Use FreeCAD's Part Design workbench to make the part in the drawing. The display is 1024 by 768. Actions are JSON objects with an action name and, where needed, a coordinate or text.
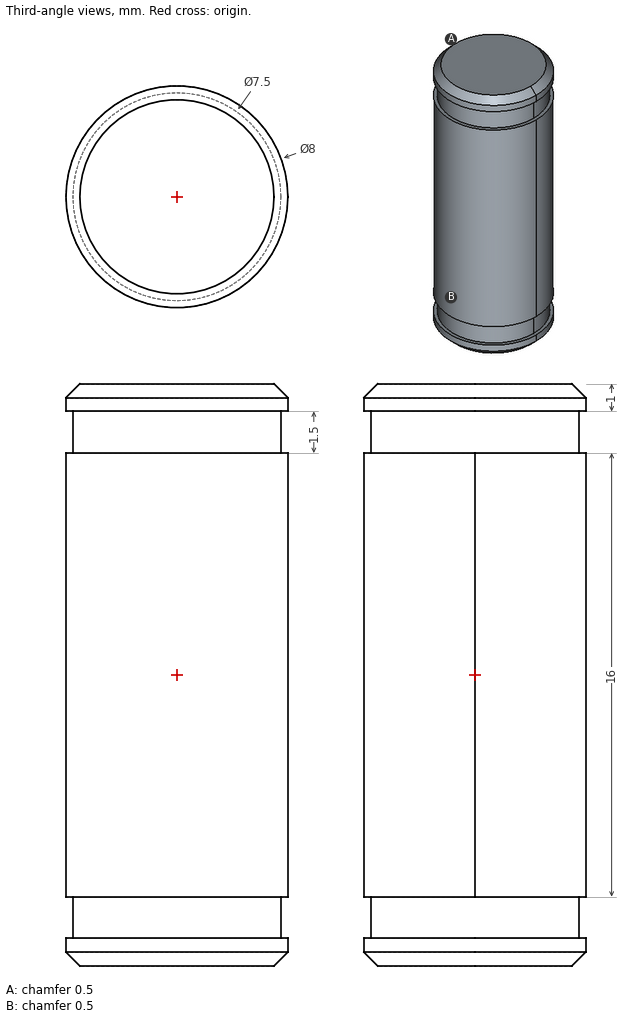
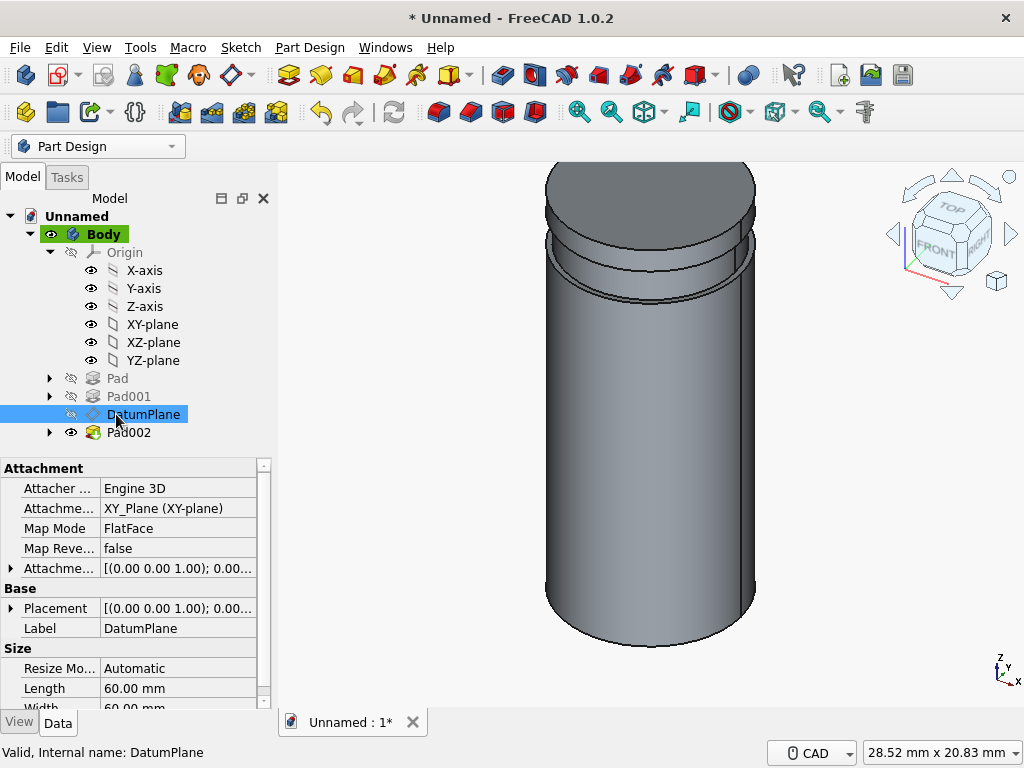
{"action": "key", "text": "v f"}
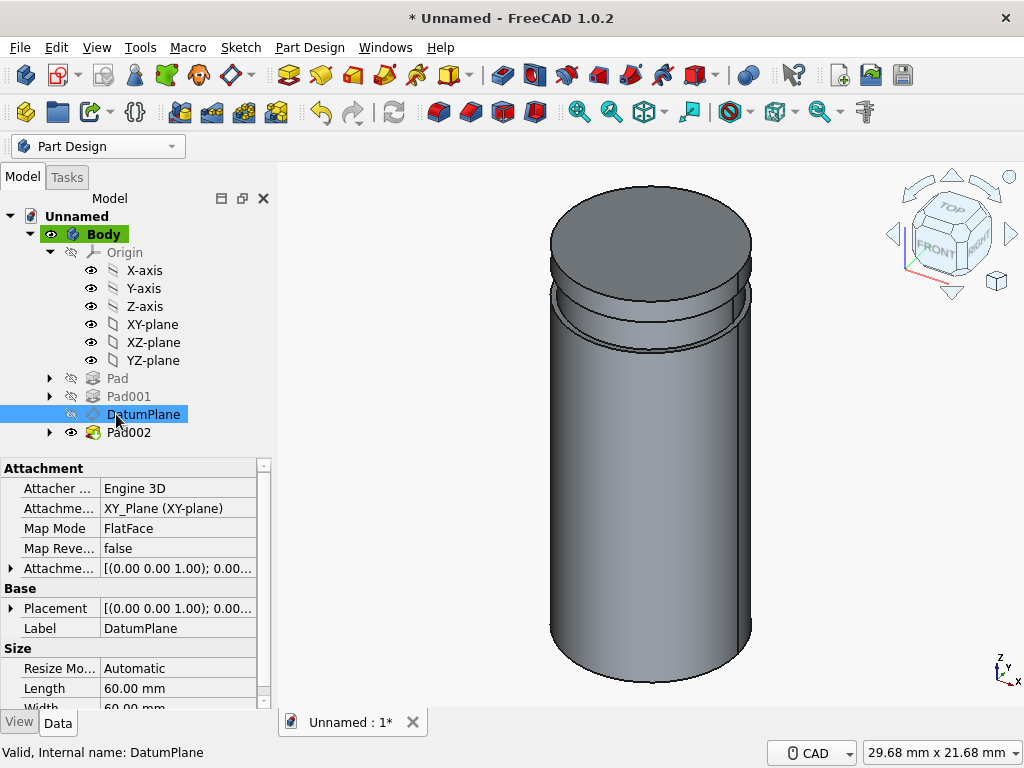
{"action": "left_click", "coordinate": [551, 249]}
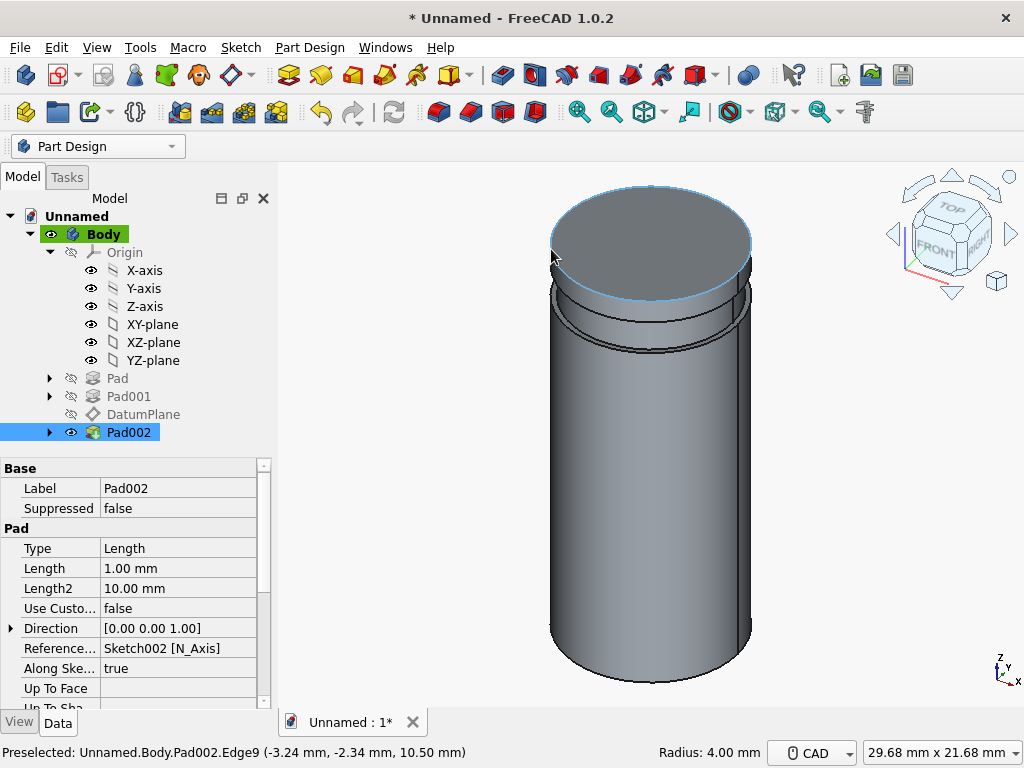
{"action": "left_click", "coordinate": [472, 112]}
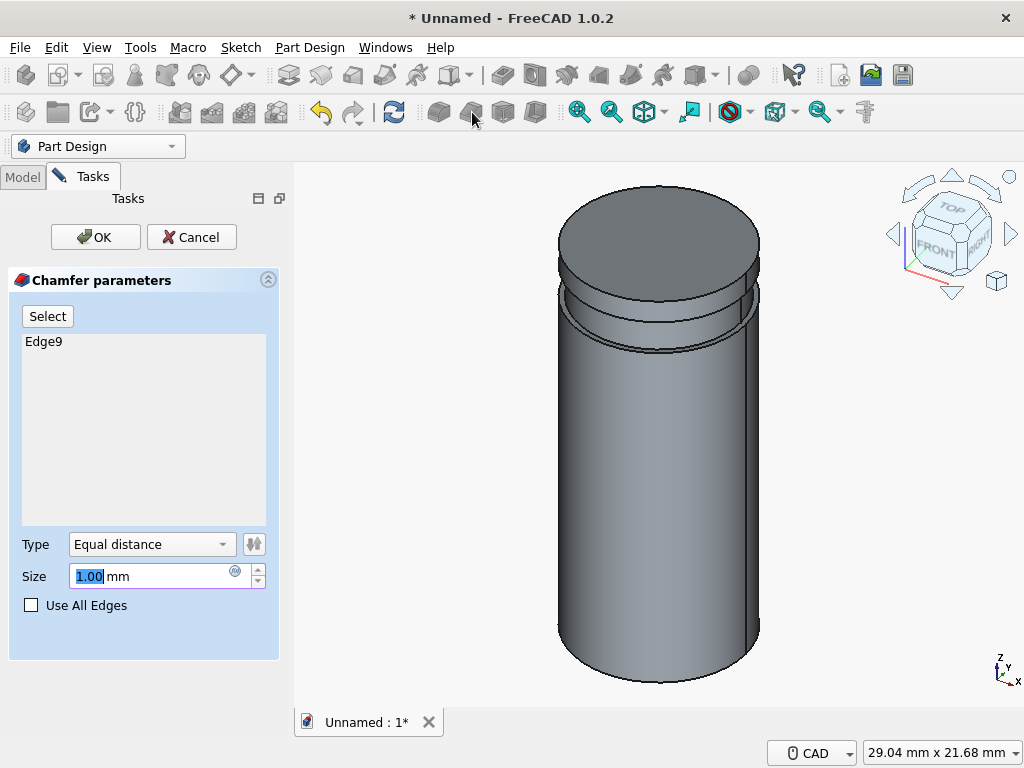
{"action": "type", "text": "0.5"}
{"action": "key", "text": "Tab"}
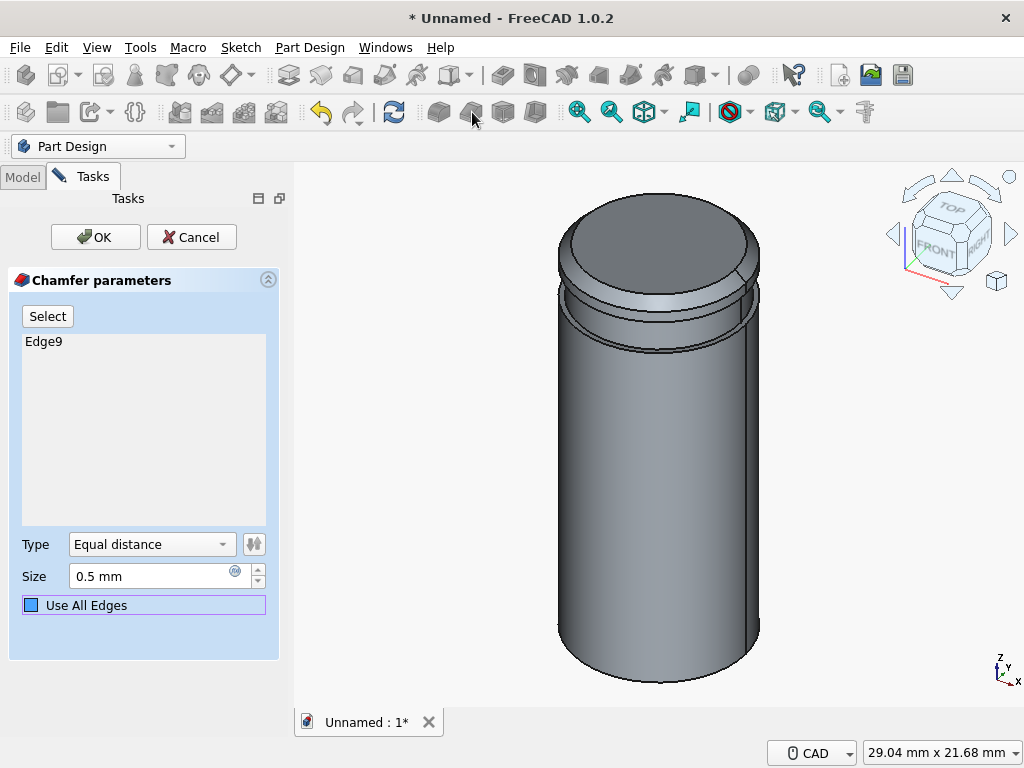
{"action": "left_click", "coordinate": [96, 237]}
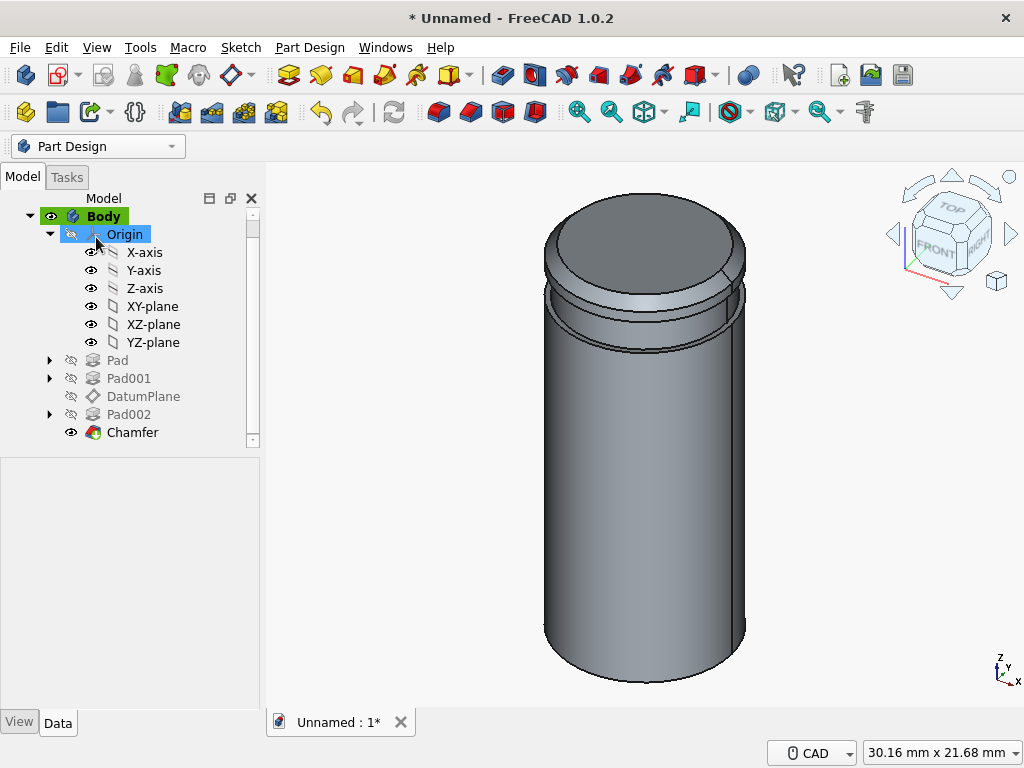
{"action": "left_click", "coordinate": [116, 378]}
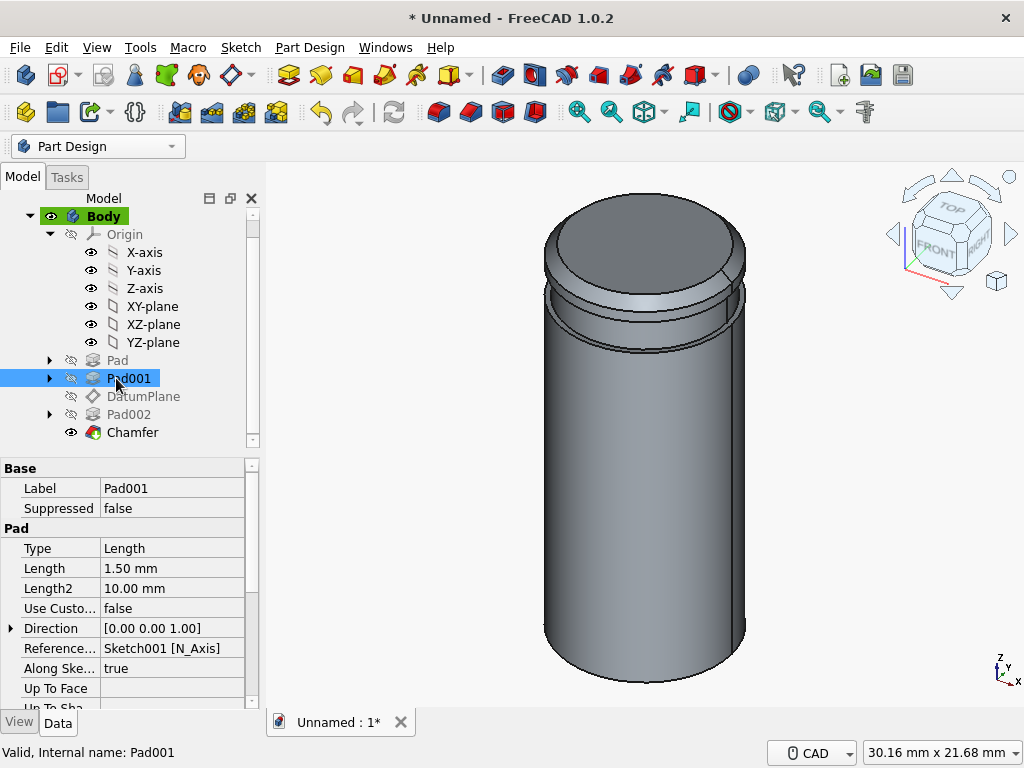
{"action": "left_click", "coordinate": [116, 414], "text": "ctrl"}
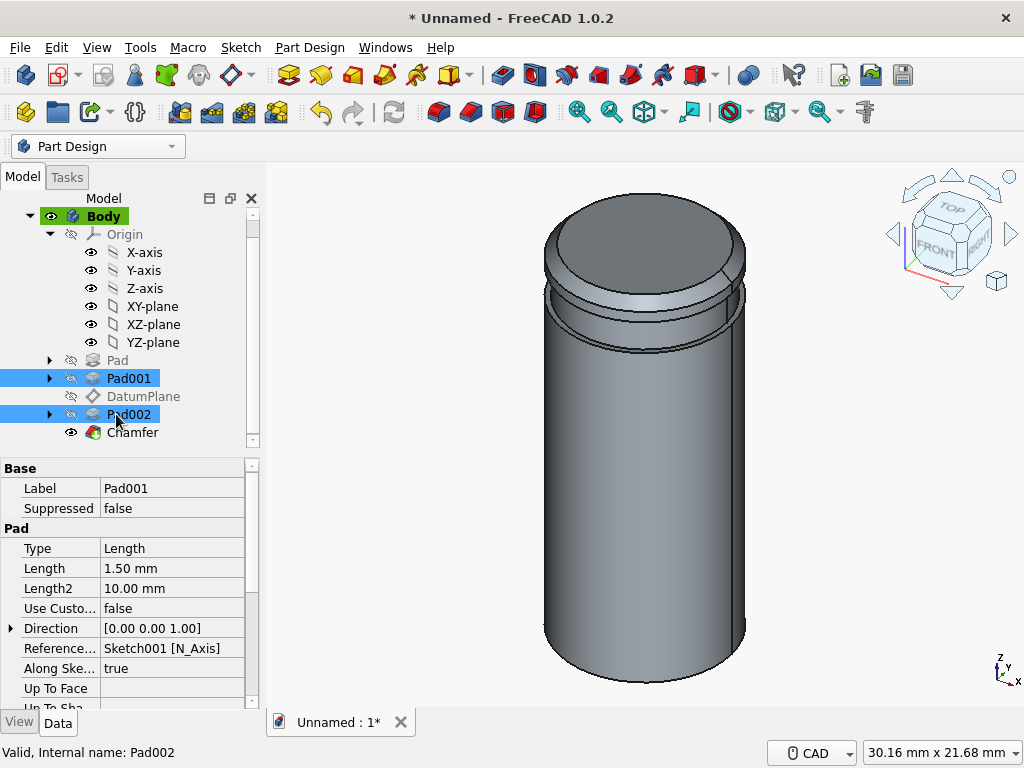
{"action": "left_click", "coordinate": [180, 112]}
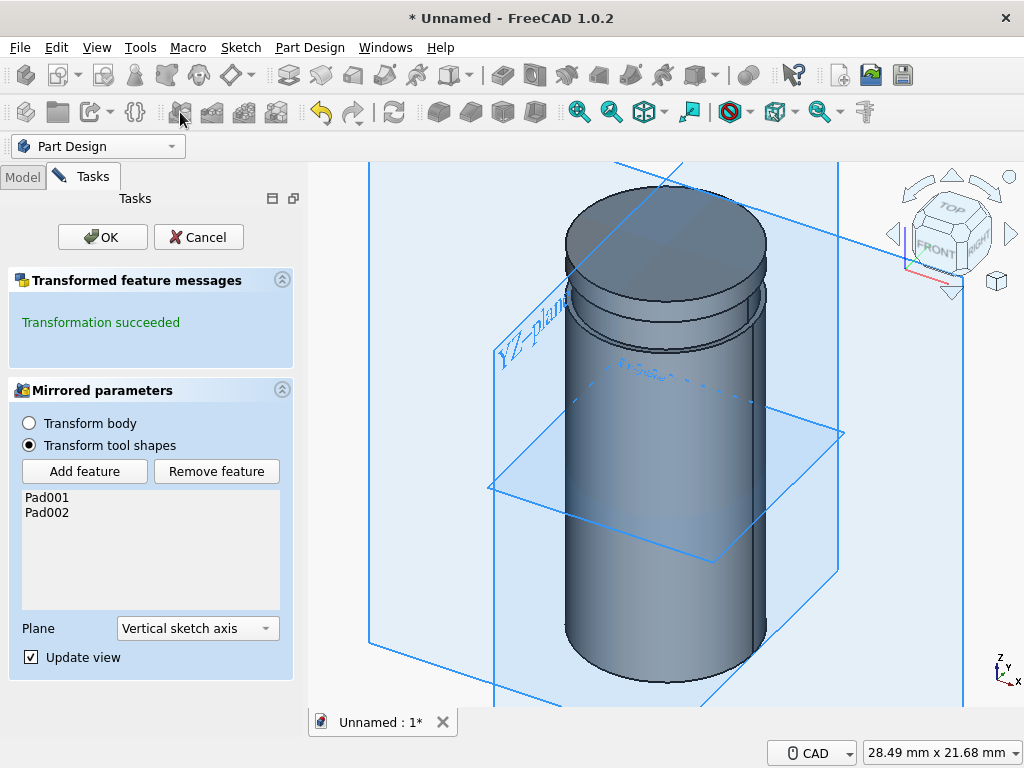
{"action": "left_click", "coordinate": [198, 628]}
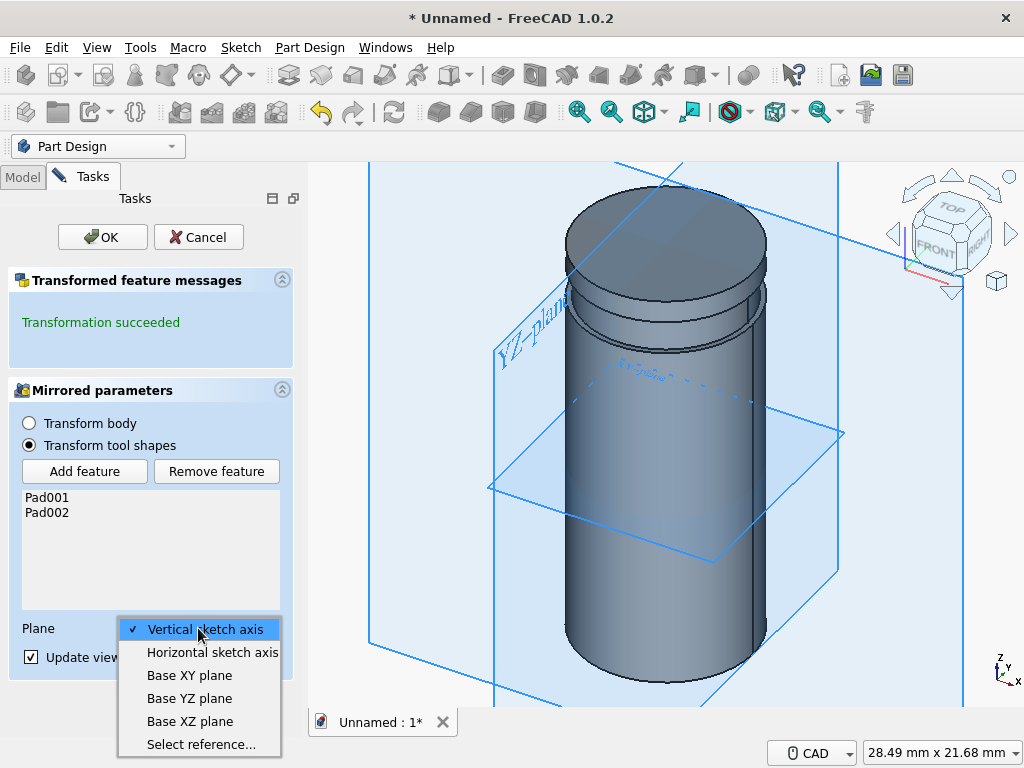
{"action": "left_click", "coordinate": [198, 676]}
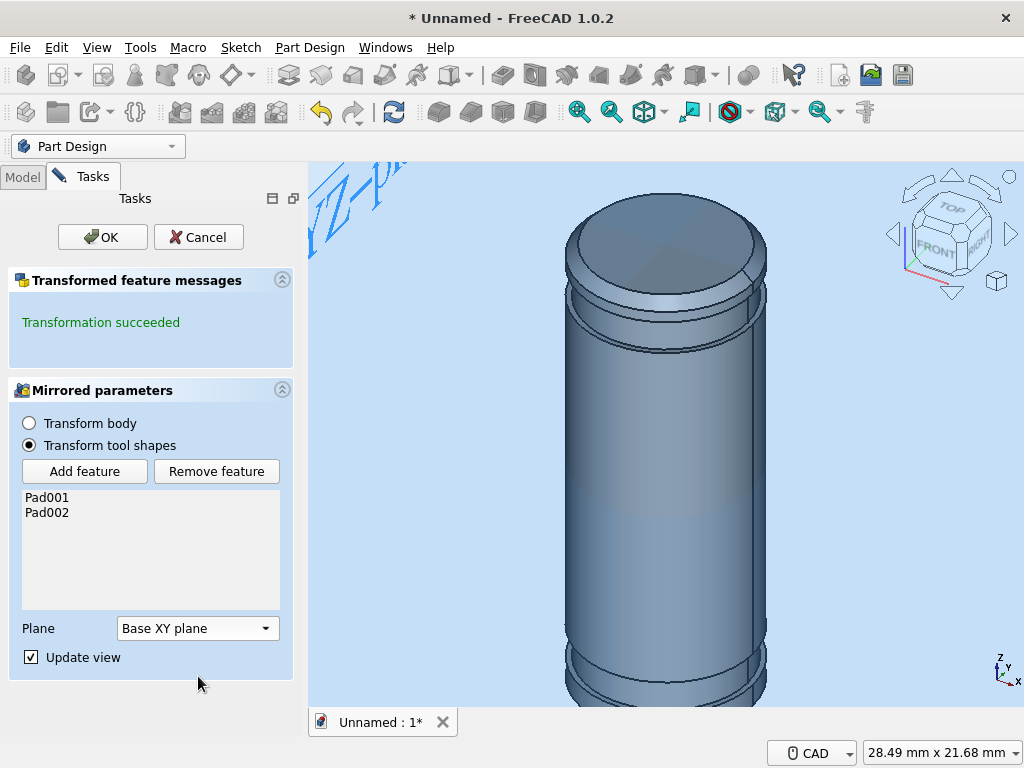
{"action": "left_click", "coordinate": [103, 237]}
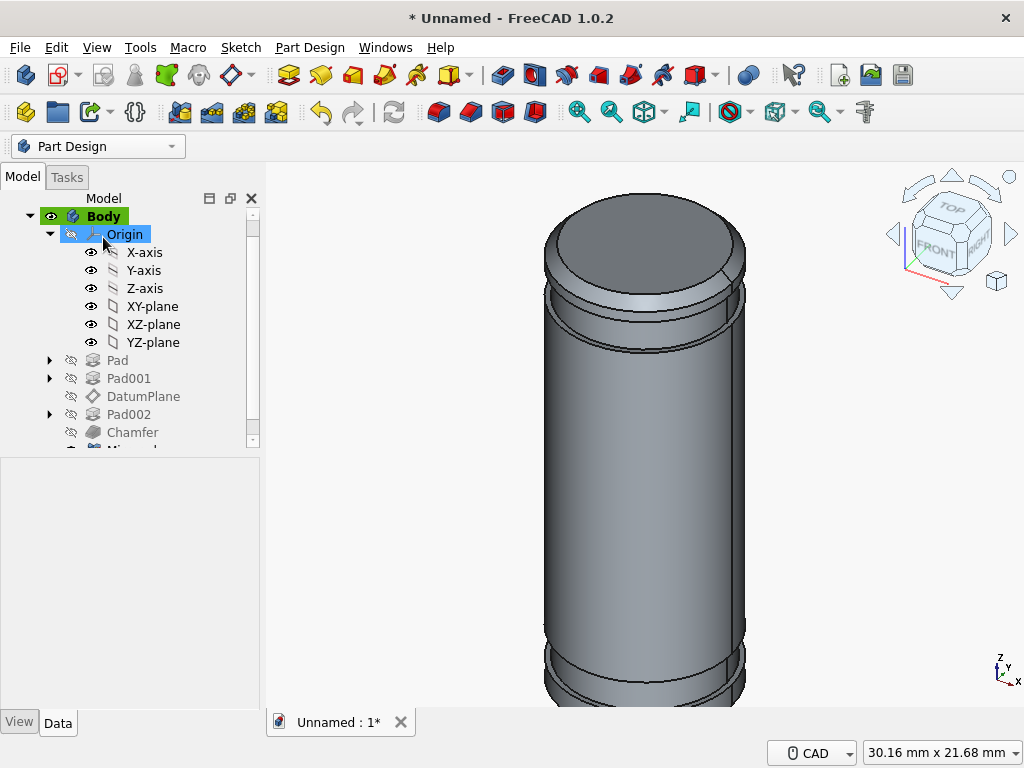
{"action": "left_click", "coordinate": [580, 112]}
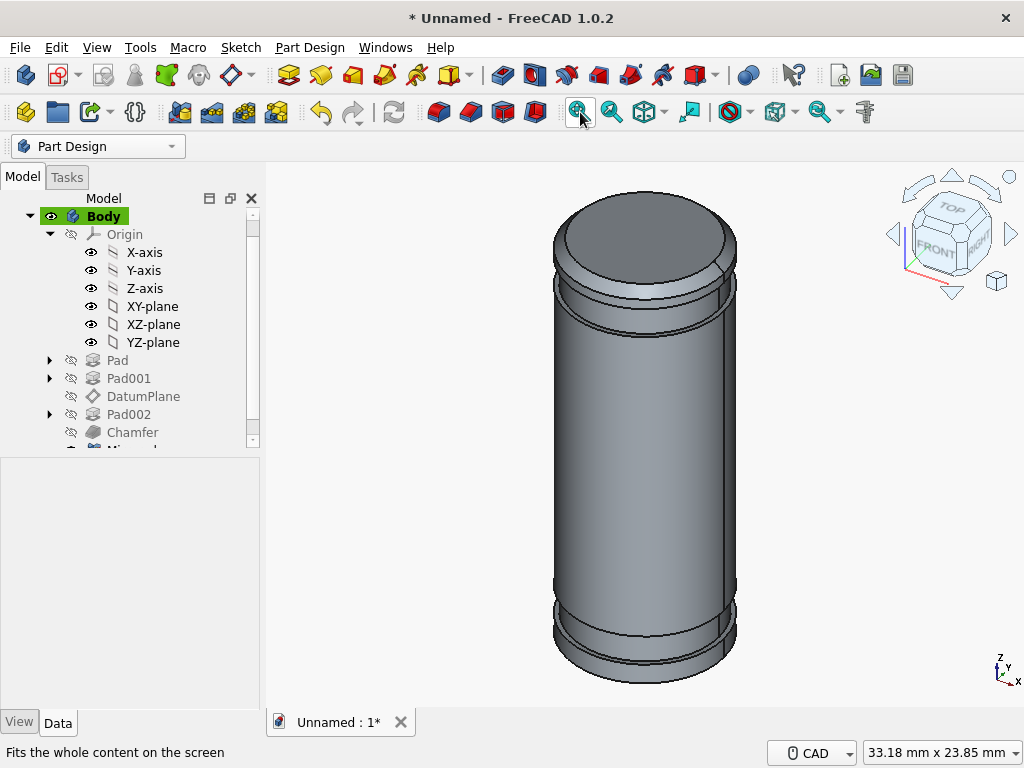
{"action": "key", "text": "0"}